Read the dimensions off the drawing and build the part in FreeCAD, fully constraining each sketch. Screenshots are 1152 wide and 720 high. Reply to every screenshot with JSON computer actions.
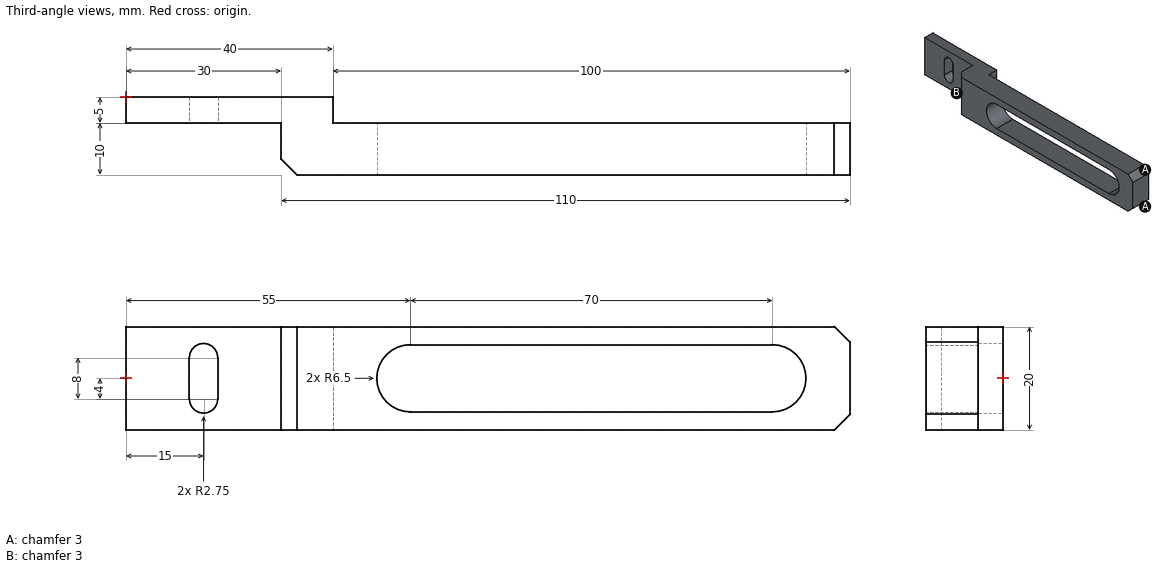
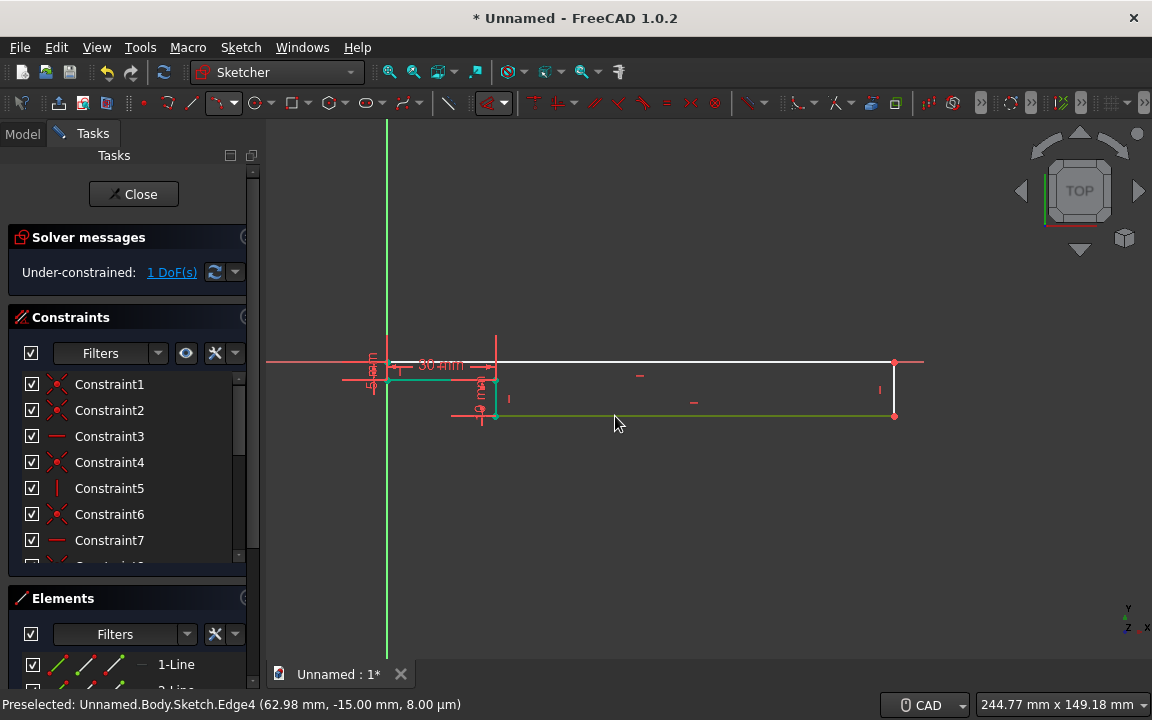
{"action": "key", "text": "l"}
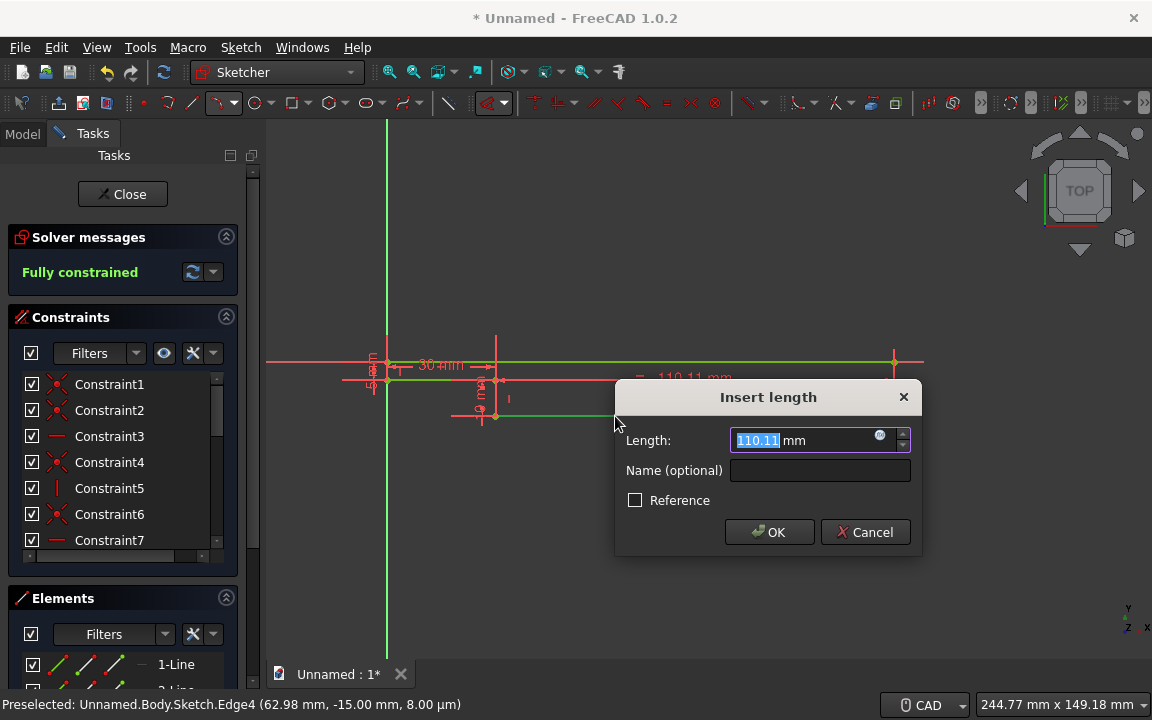
{"action": "type", "text": "110"}
{"action": "key", "text": "Return"}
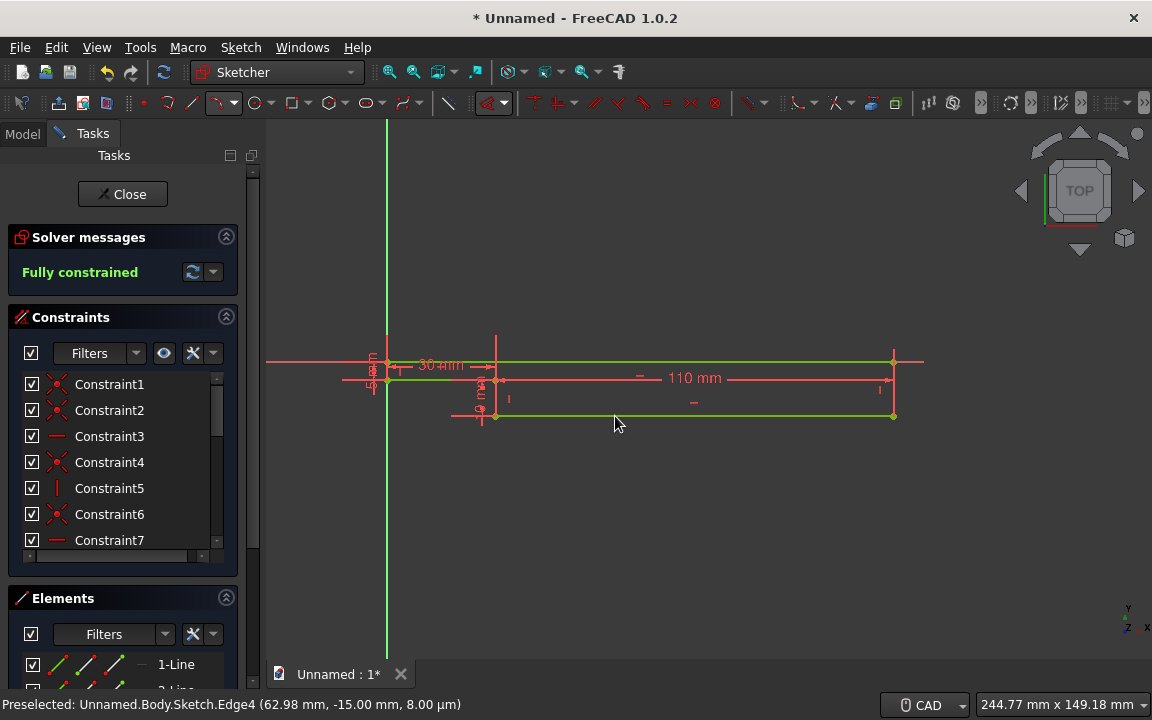
{"action": "left_click", "coordinate": [123, 194]}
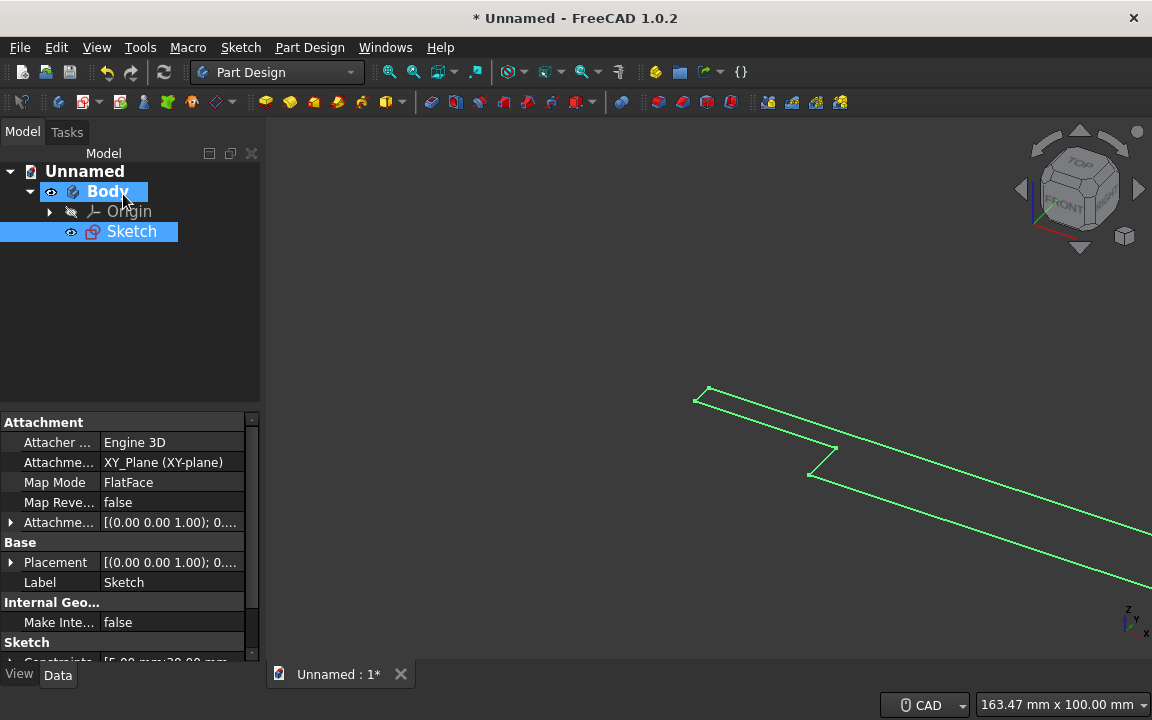
{"action": "left_click", "coordinate": [266, 102]}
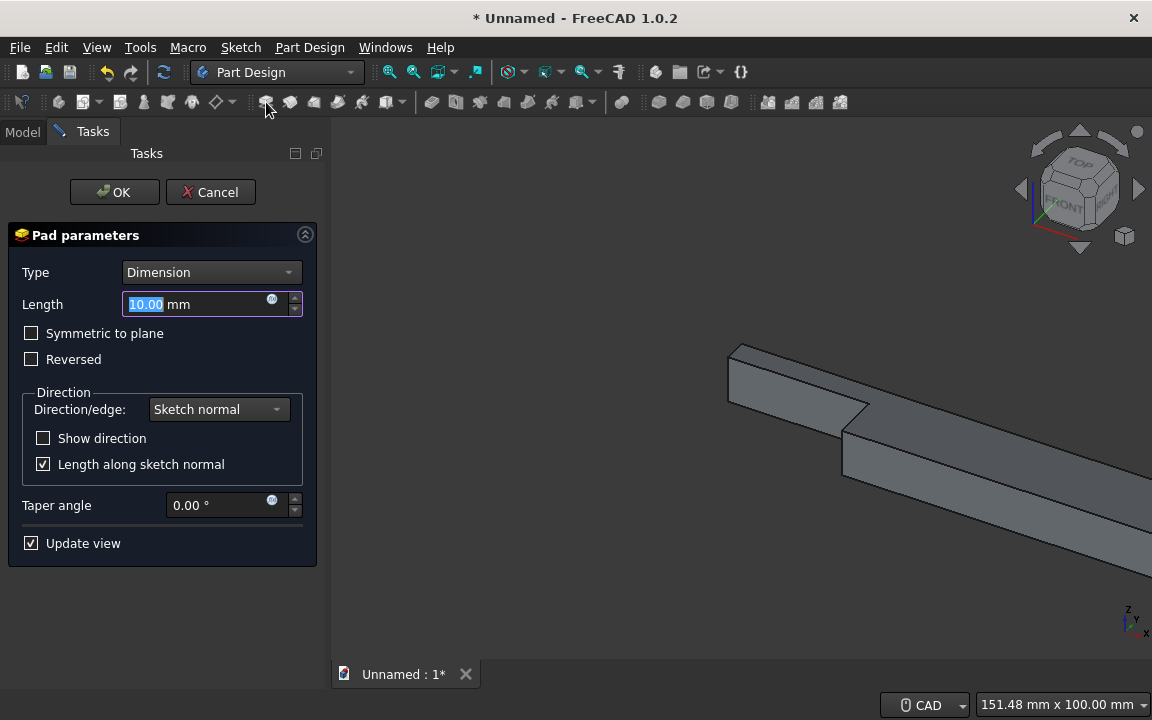
{"action": "type", "text": "20"}
{"action": "key", "text": "Tab"}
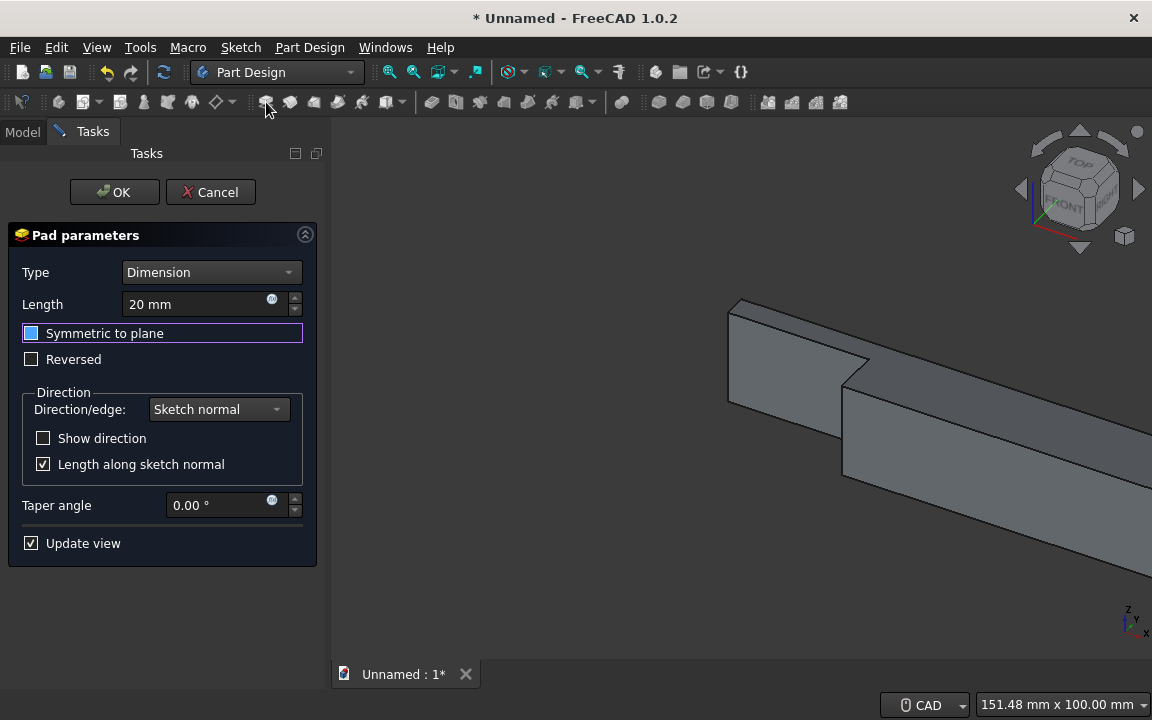
{"action": "left_click", "coordinate": [30, 333]}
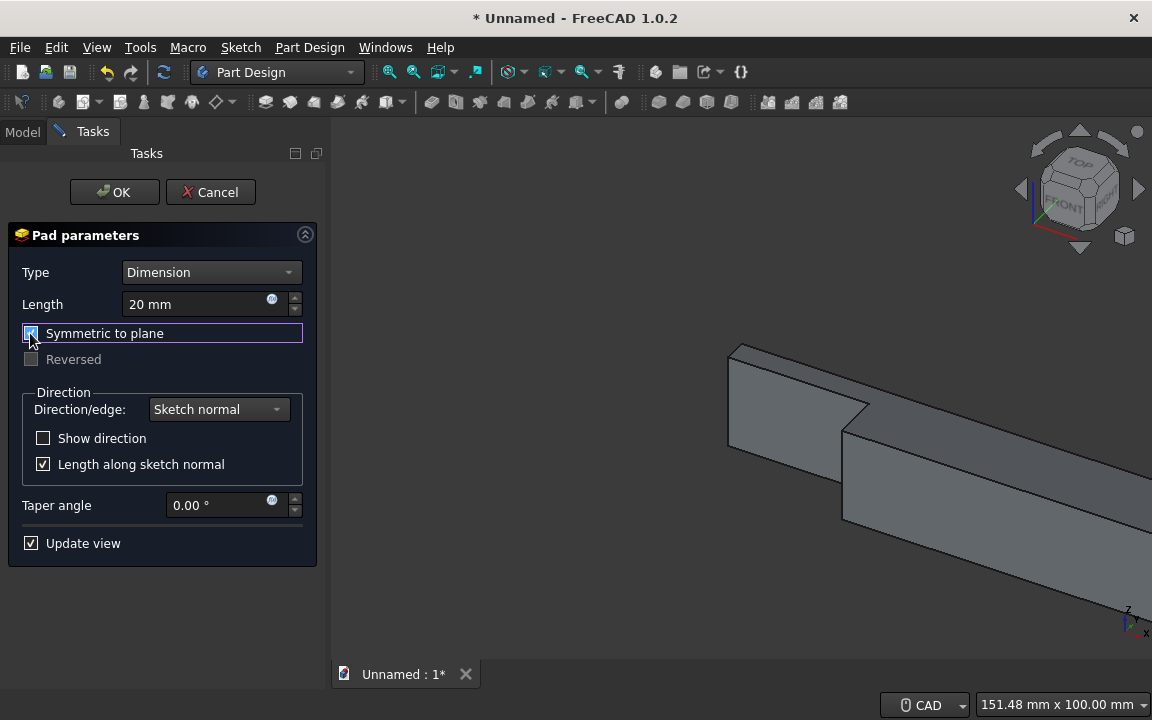
{"action": "left_click", "coordinate": [115, 192]}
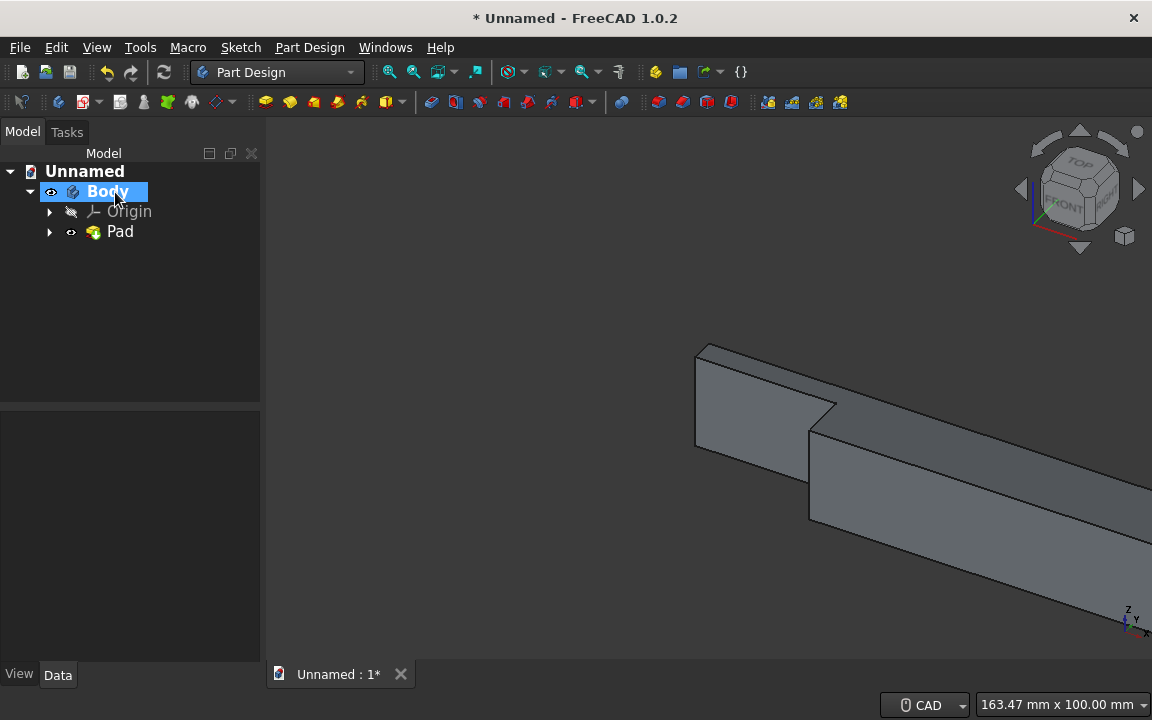
{"action": "left_click", "coordinate": [390, 72]}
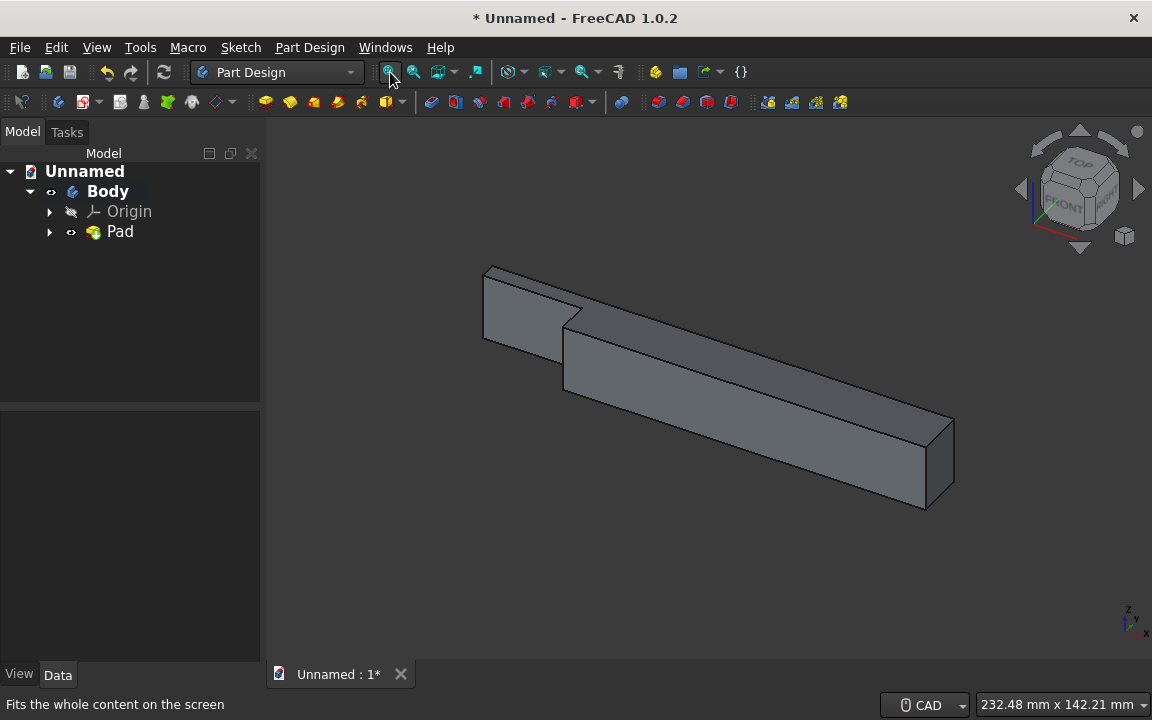
{"action": "left_click", "coordinate": [84, 102]}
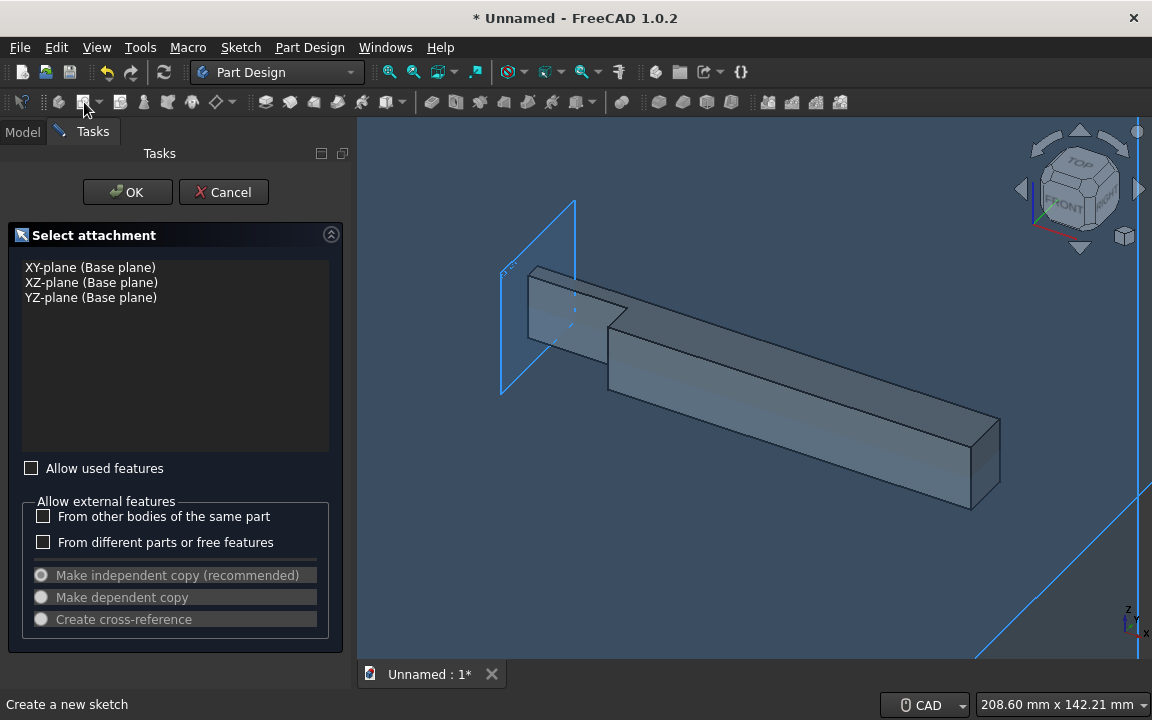
{"action": "left_click", "coordinate": [82, 282]}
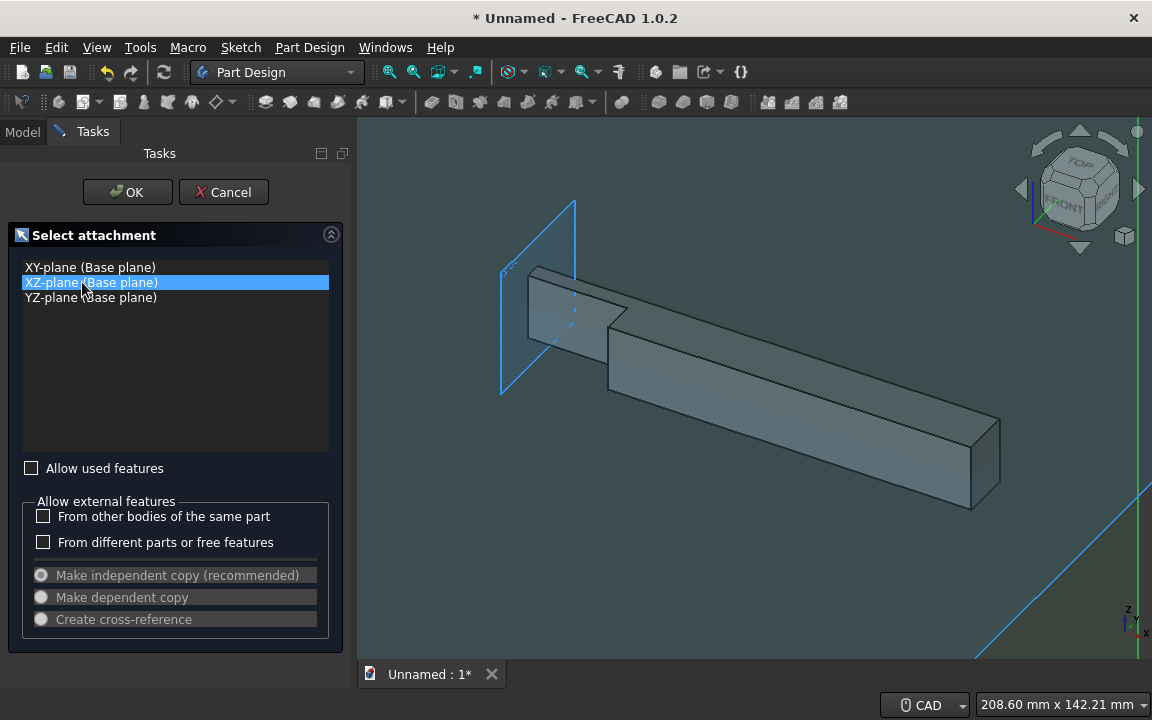
{"action": "left_click", "coordinate": [128, 192]}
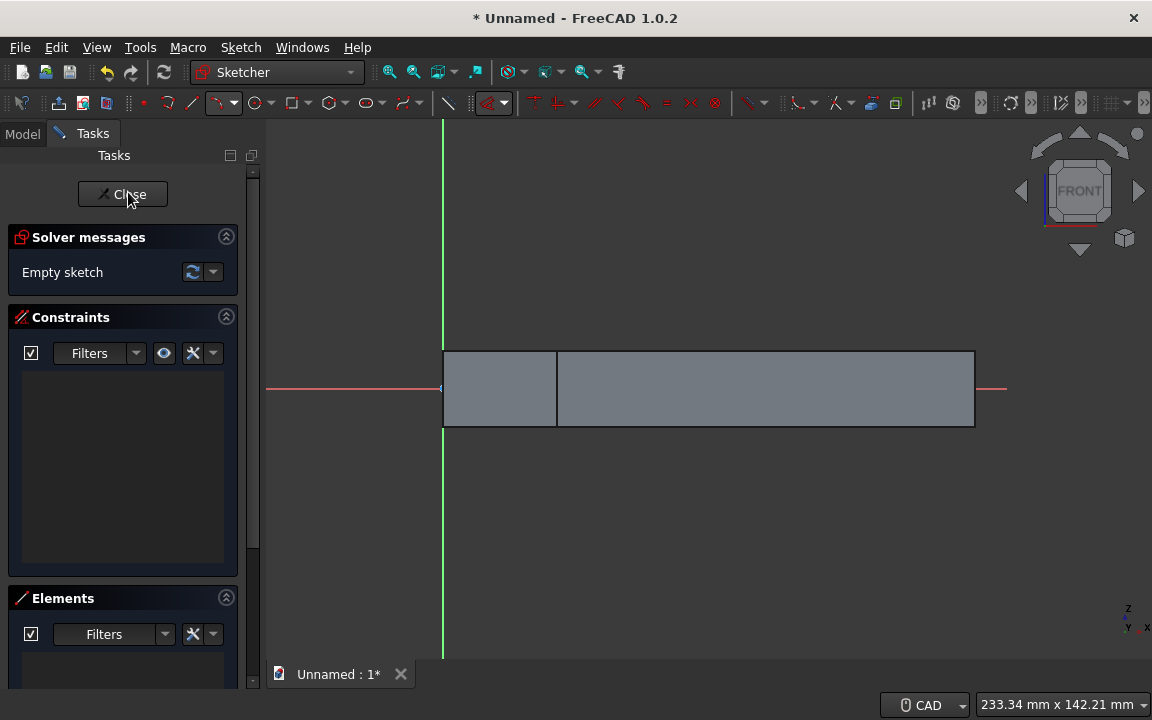
{"action": "left_click", "coordinate": [108, 104]}